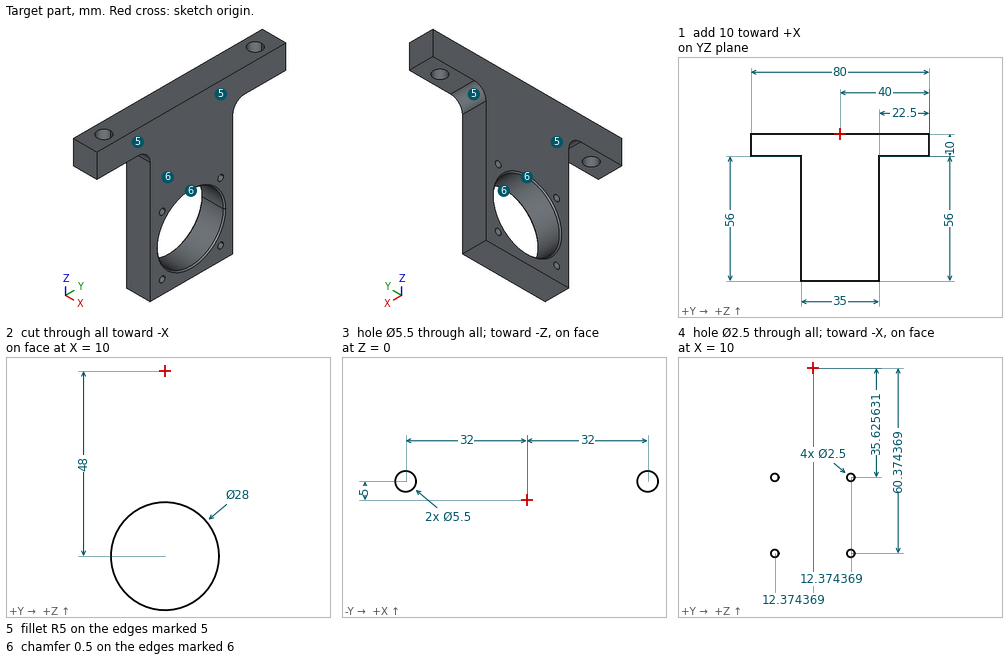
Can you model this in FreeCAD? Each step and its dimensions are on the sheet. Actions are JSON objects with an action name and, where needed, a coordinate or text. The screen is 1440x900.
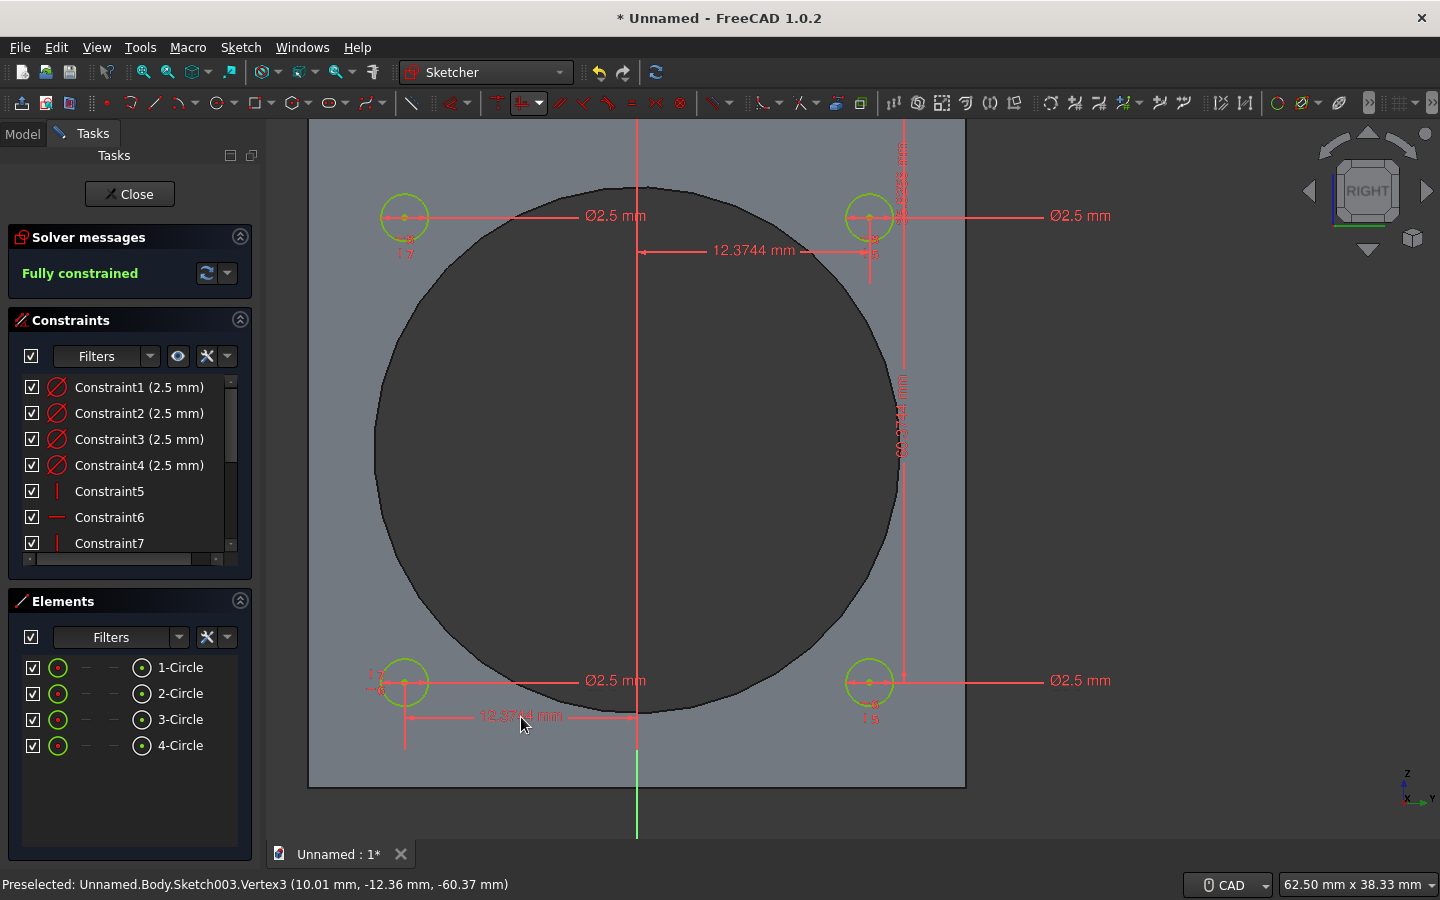
{"action": "left_click", "coordinate": [130, 194]}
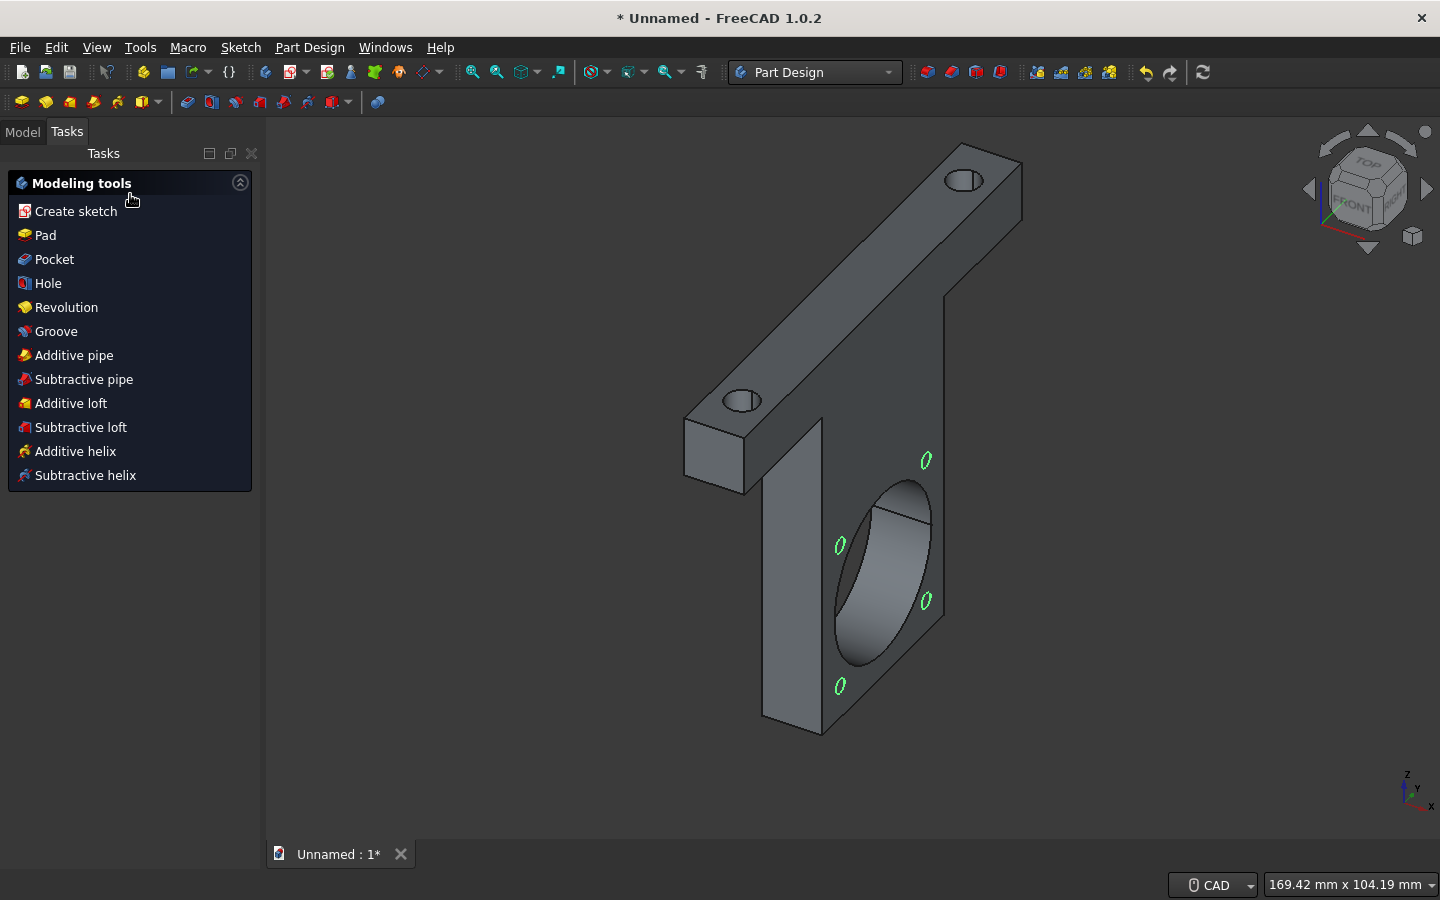
{"action": "left_click", "coordinate": [212, 102]}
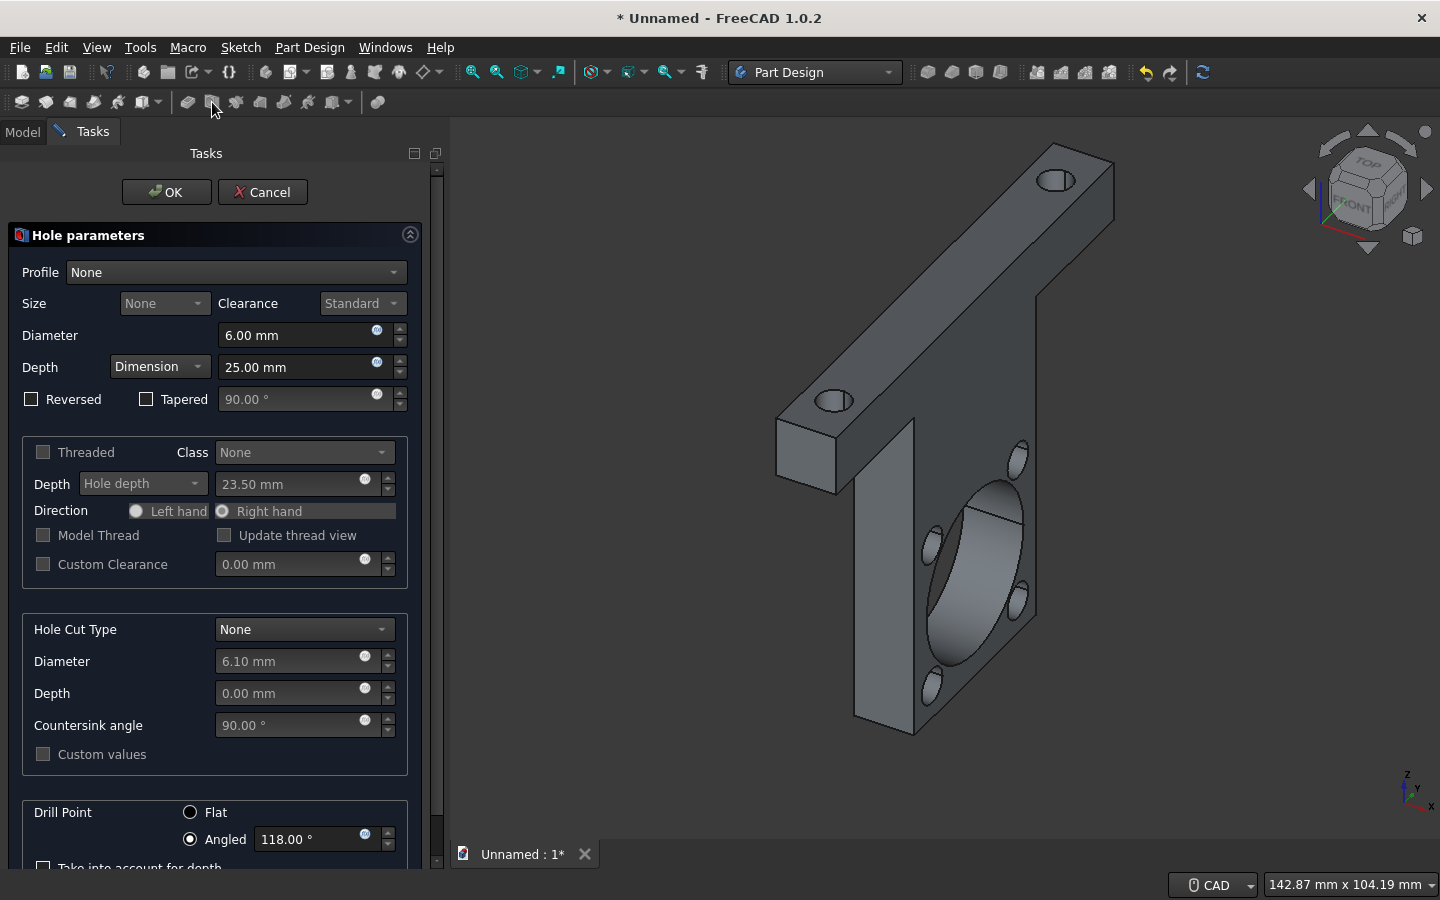
{"action": "triple_click", "coordinate": [305, 335]}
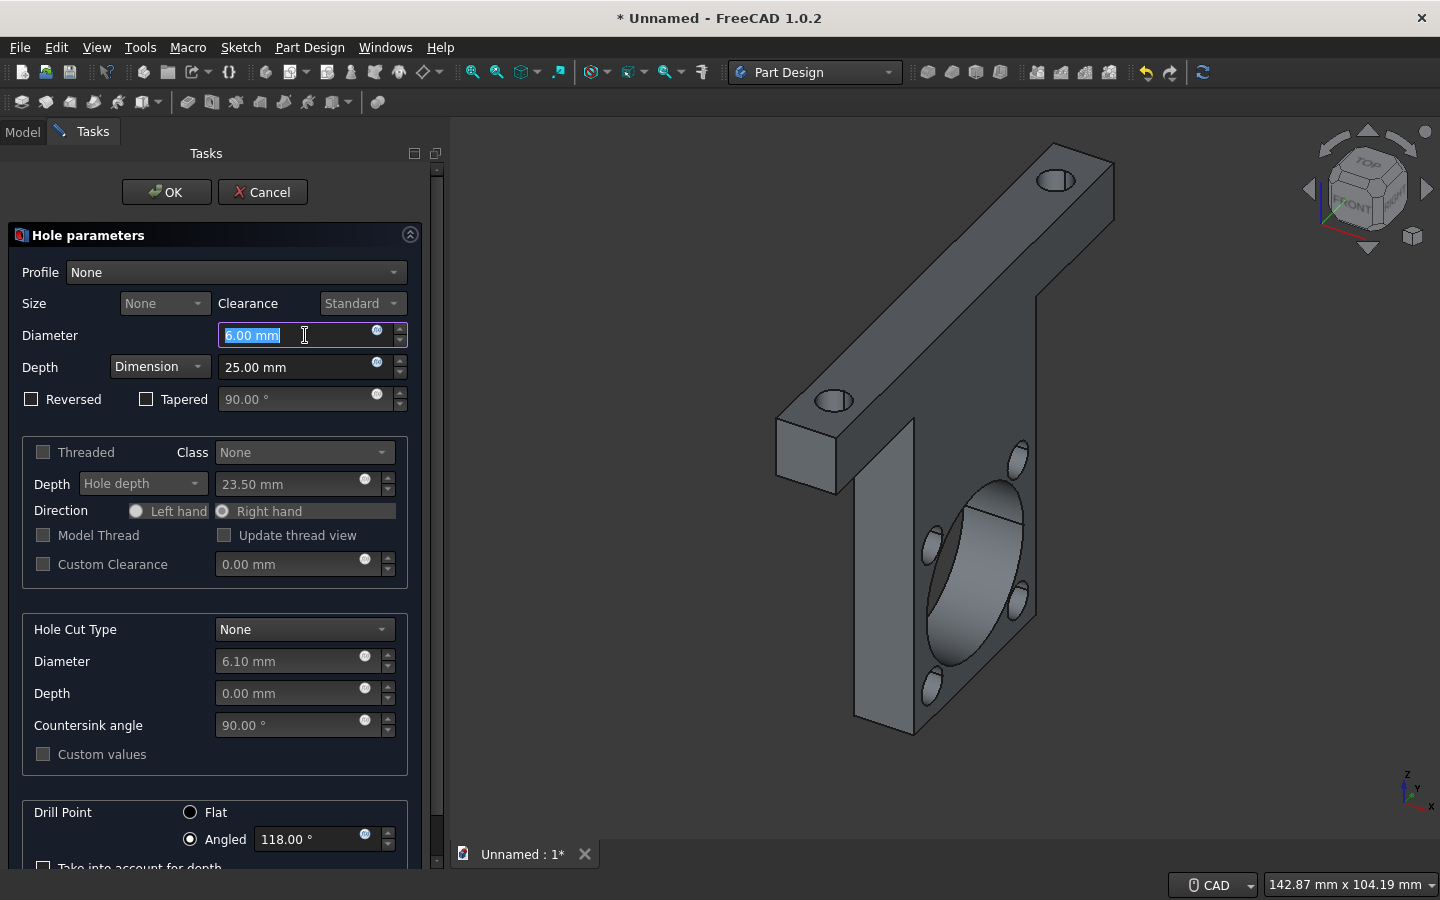
{"action": "type", "text": "2.5"}
{"action": "key", "text": "Tab"}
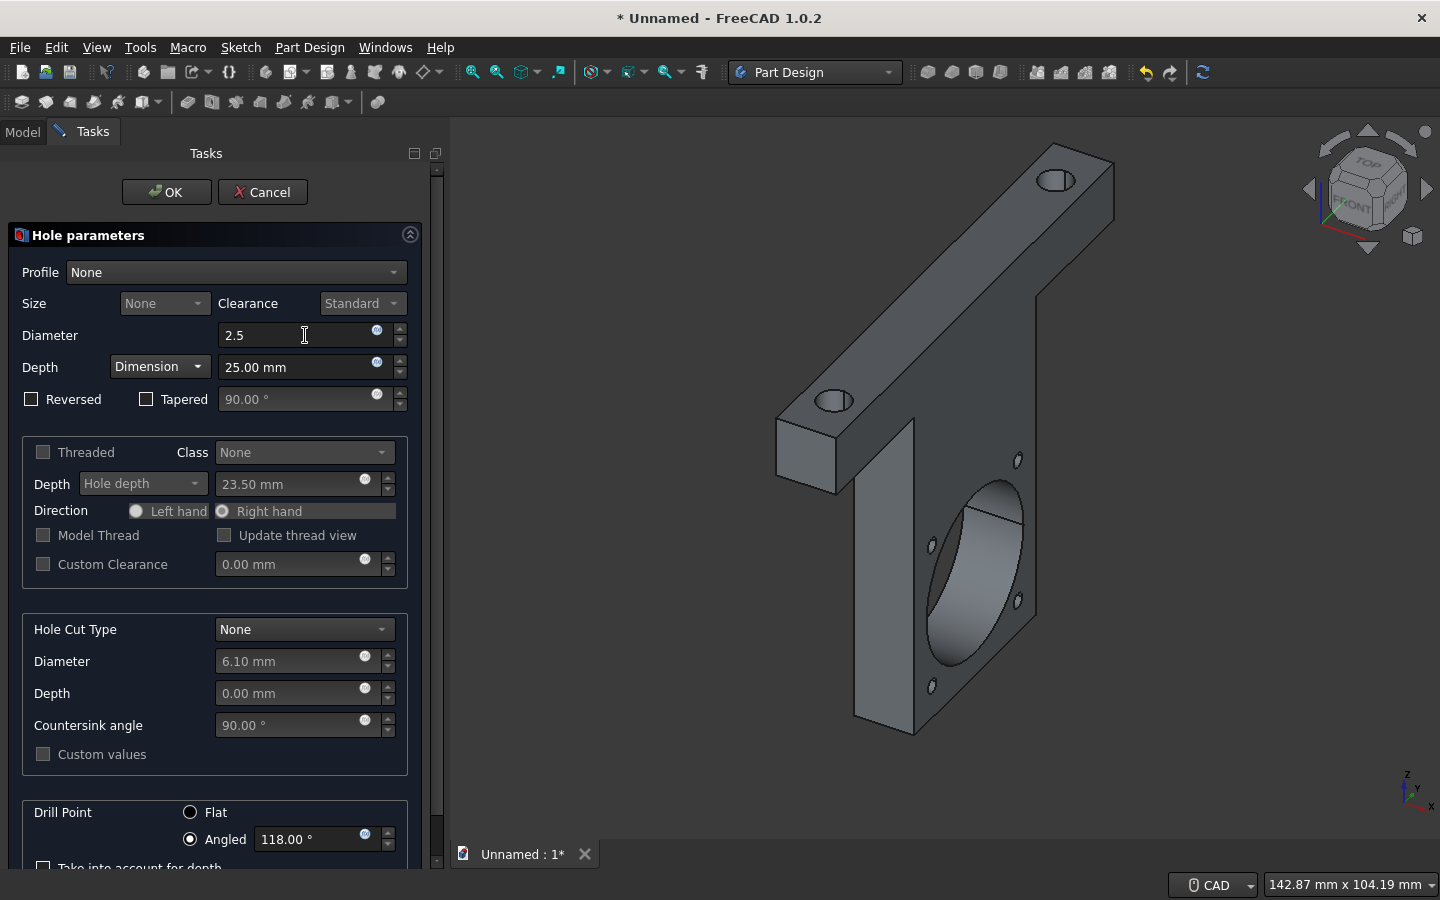
{"action": "left_click", "coordinate": [161, 366]}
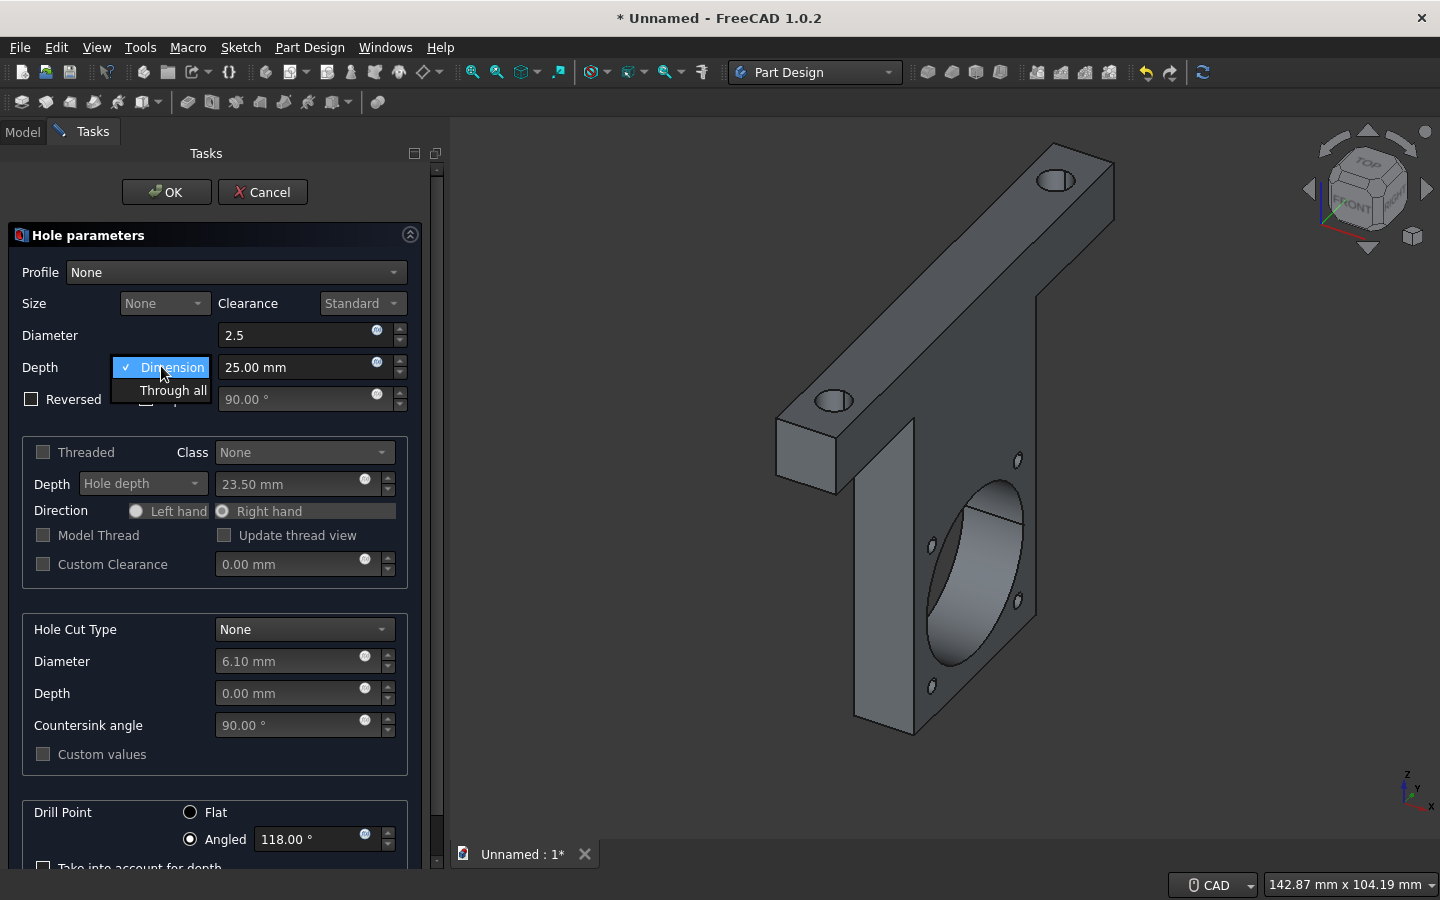
{"action": "left_click", "coordinate": [160, 390]}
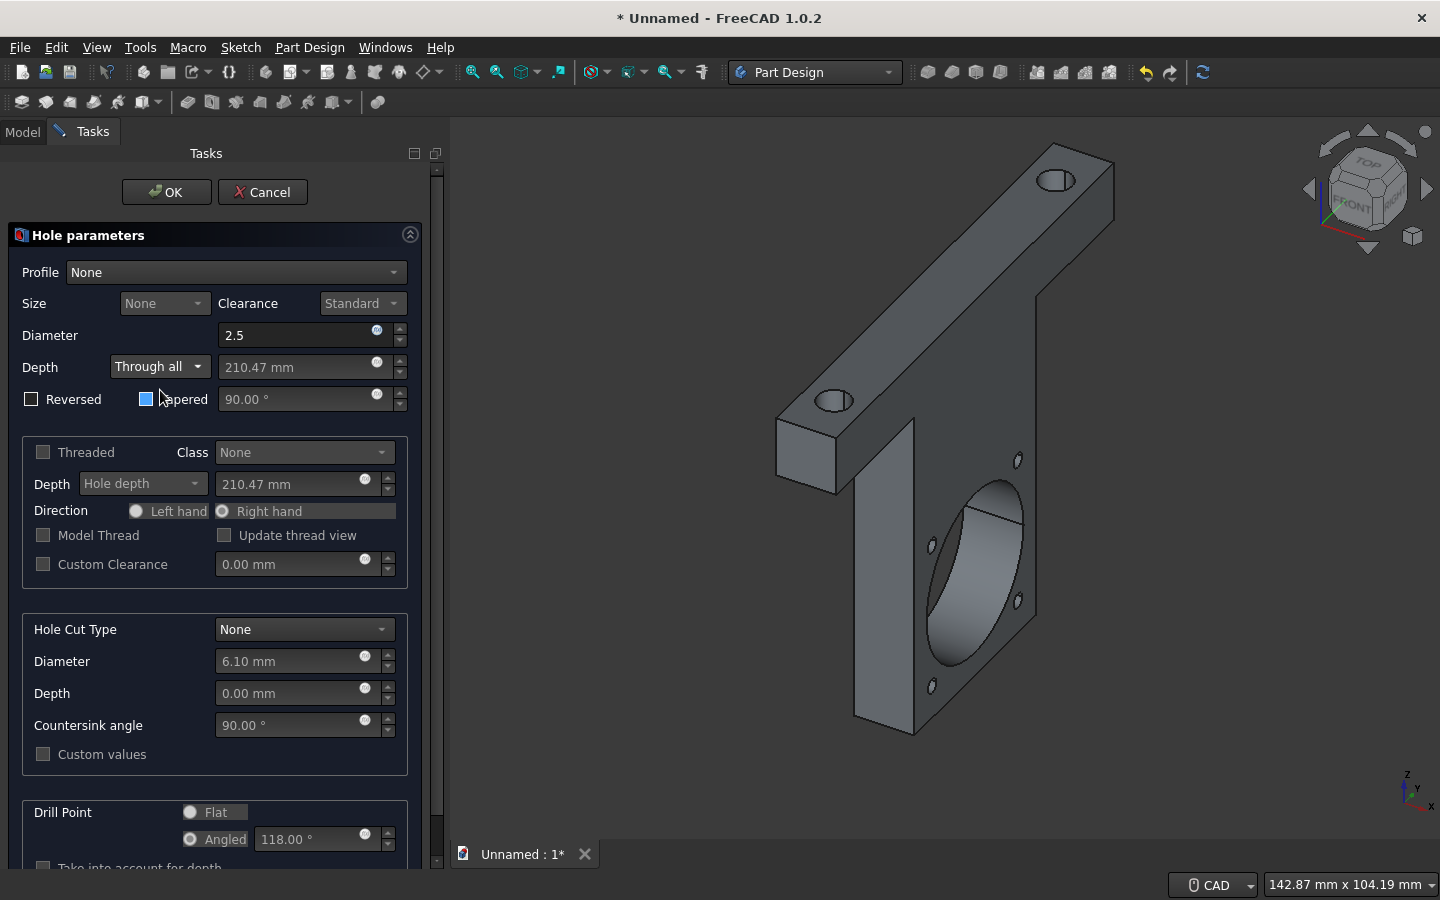
{"action": "left_click", "coordinate": [167, 192]}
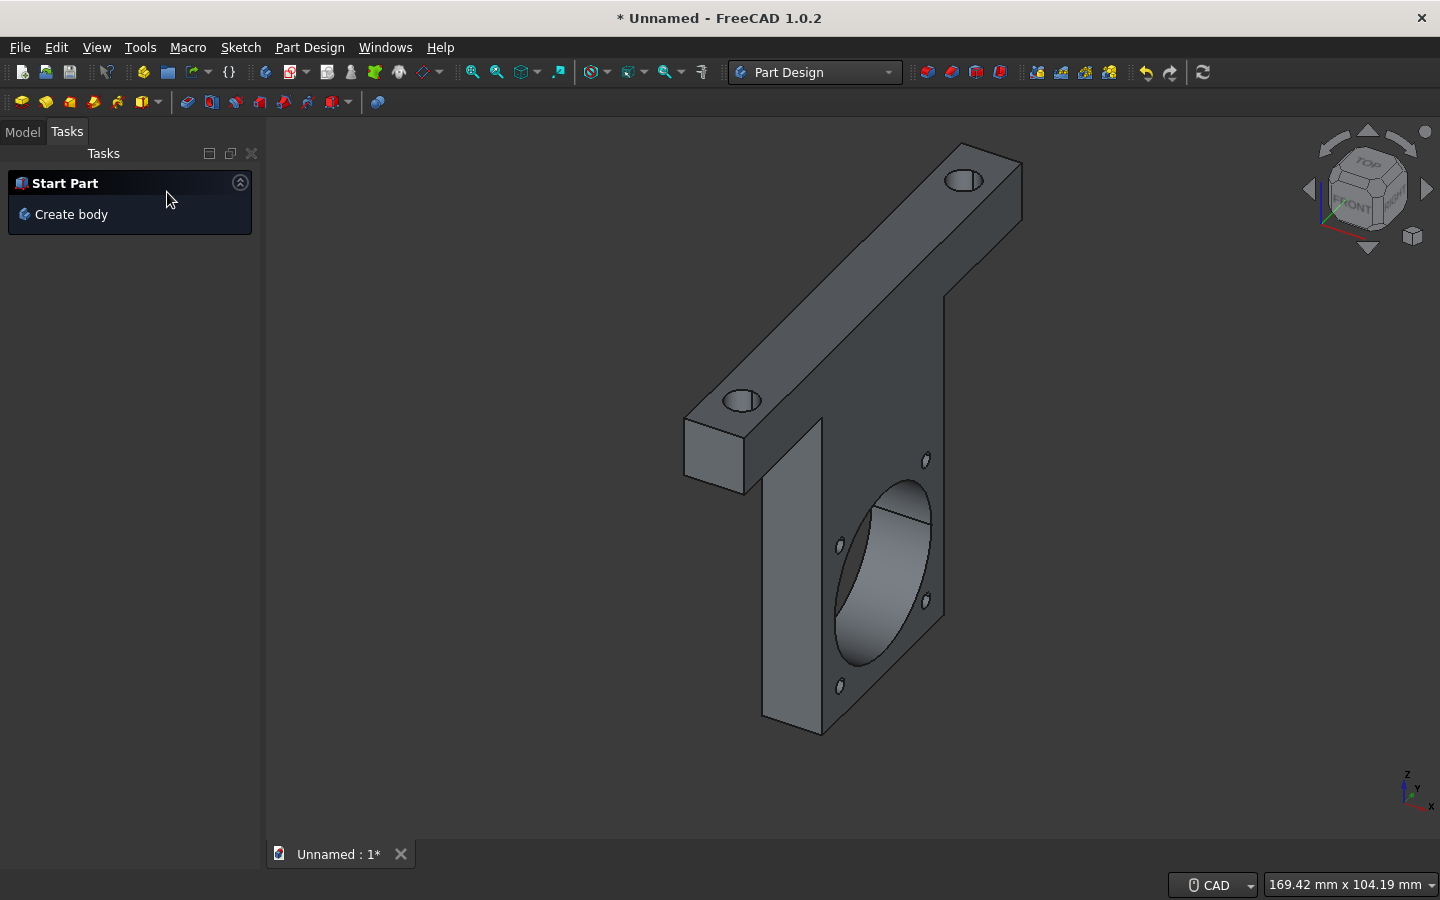
{"action": "key", "text": "0"}